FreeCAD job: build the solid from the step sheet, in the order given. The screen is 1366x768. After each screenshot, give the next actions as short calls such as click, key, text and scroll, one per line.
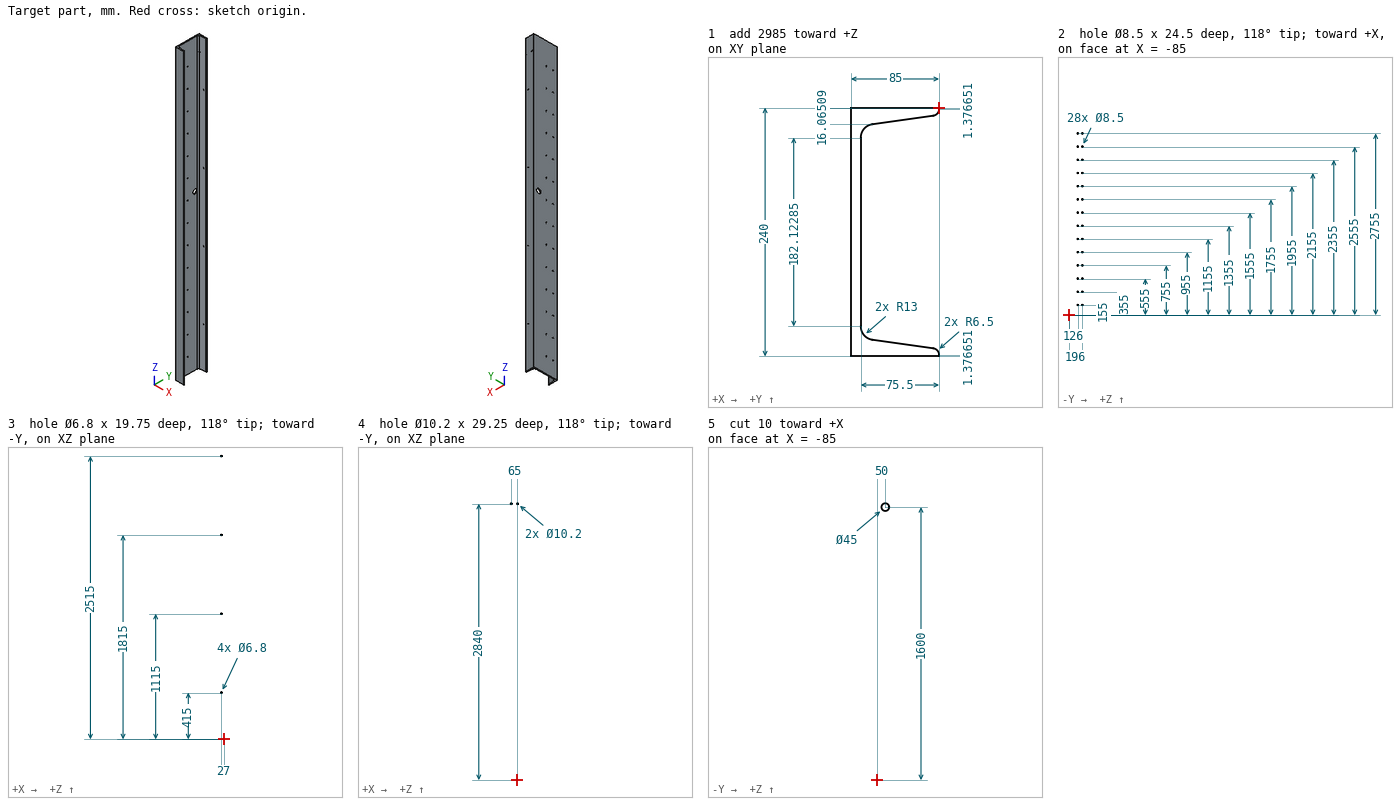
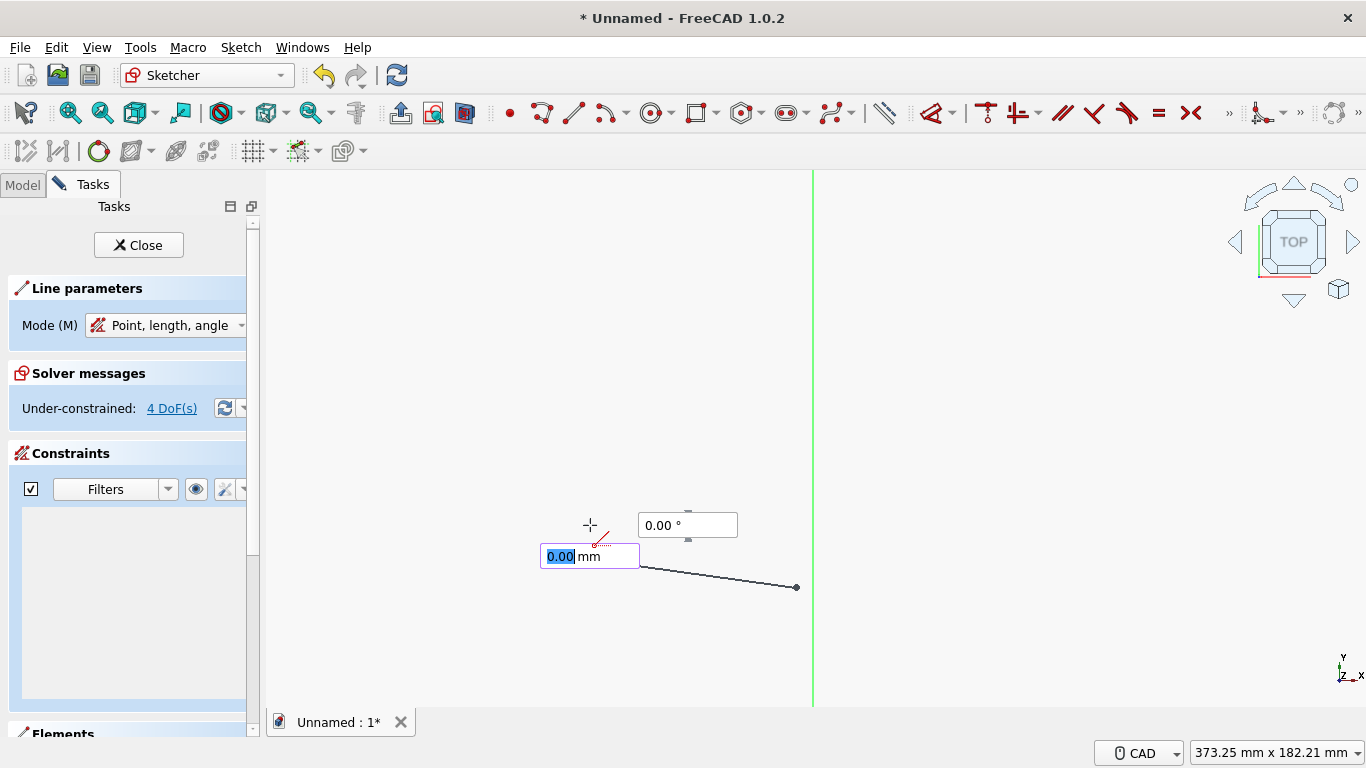
scroll(797, 587, down, 4)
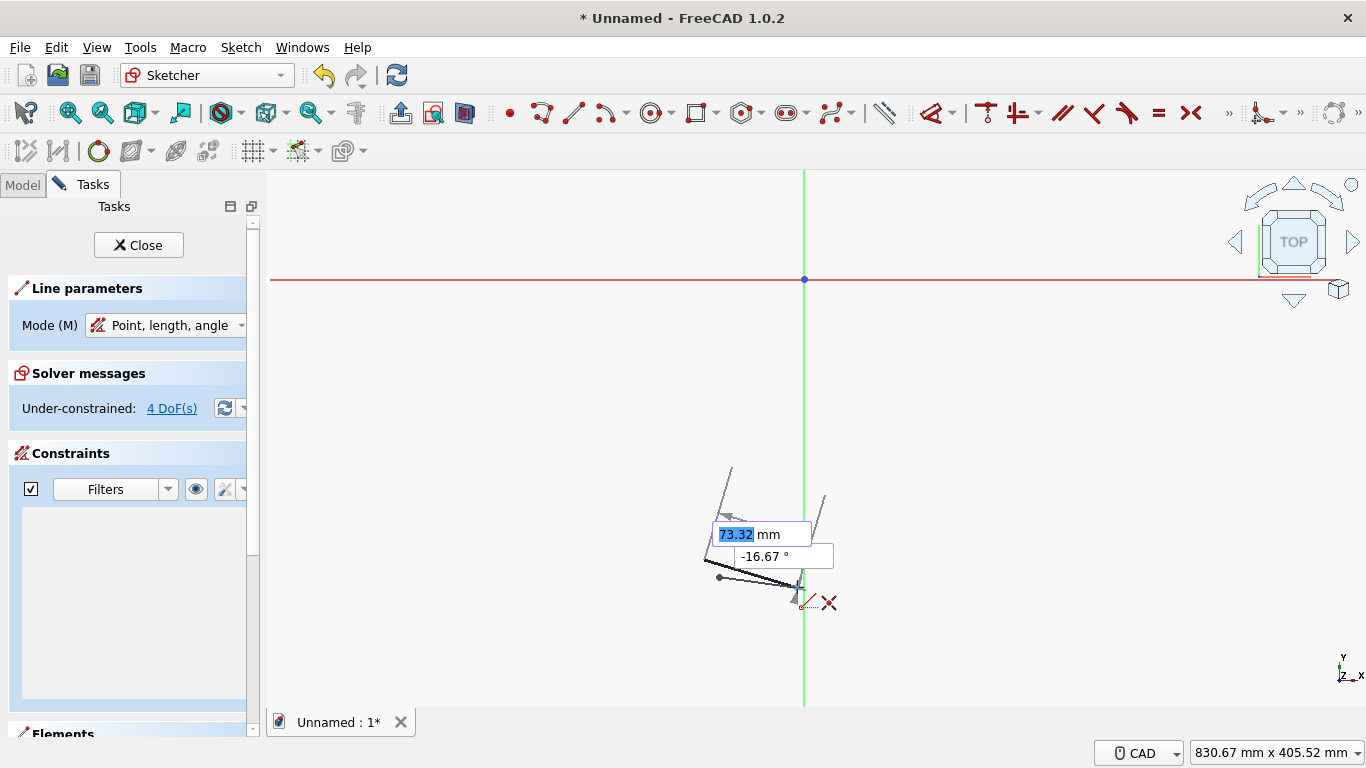
click(704, 318)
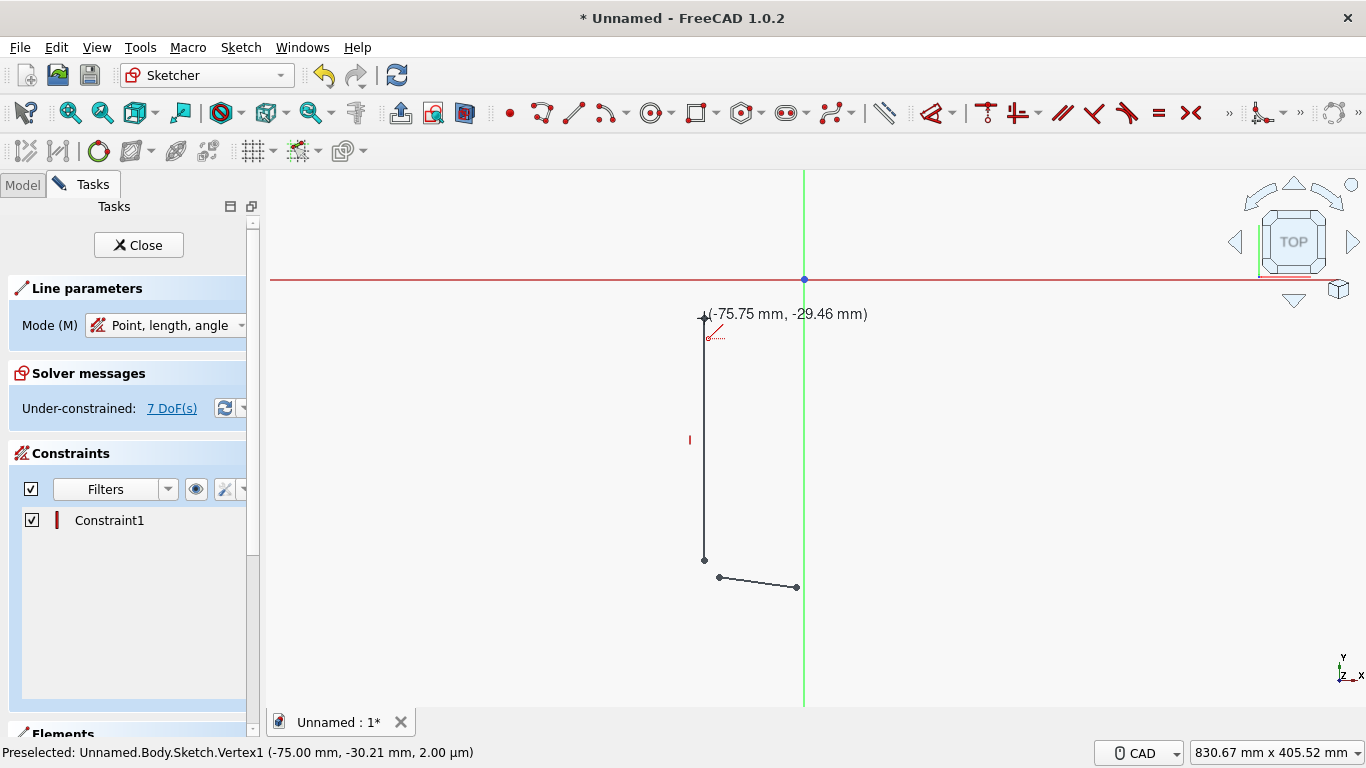
click(719, 301)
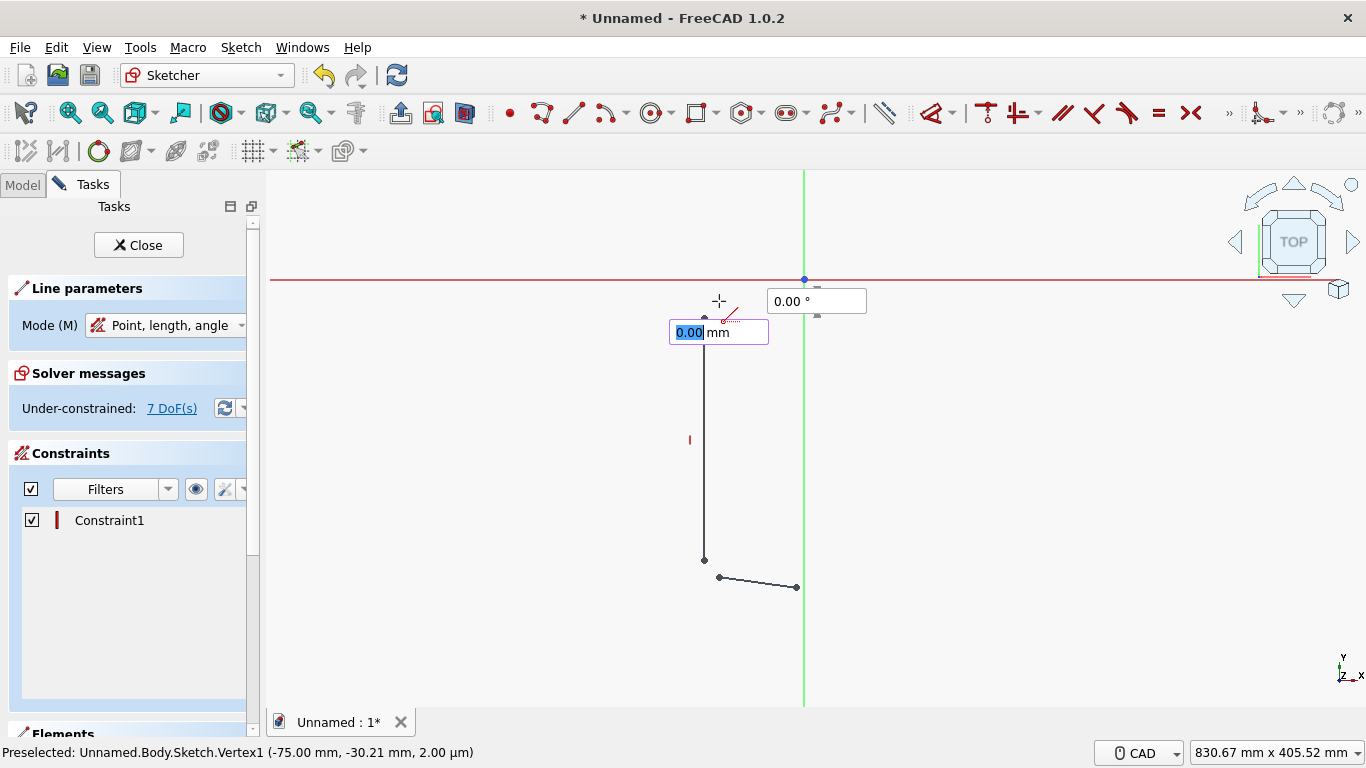
scroll(797, 290, up, 4)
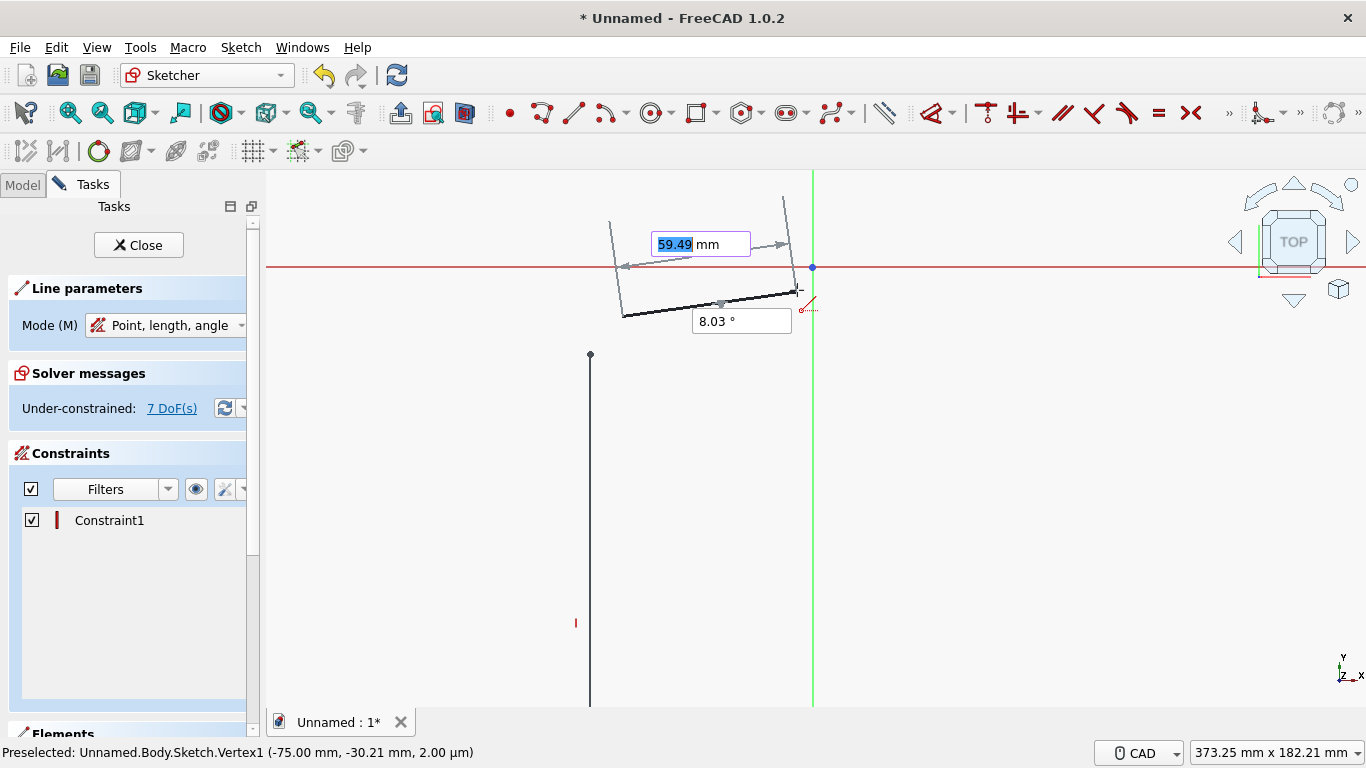
click(796, 290)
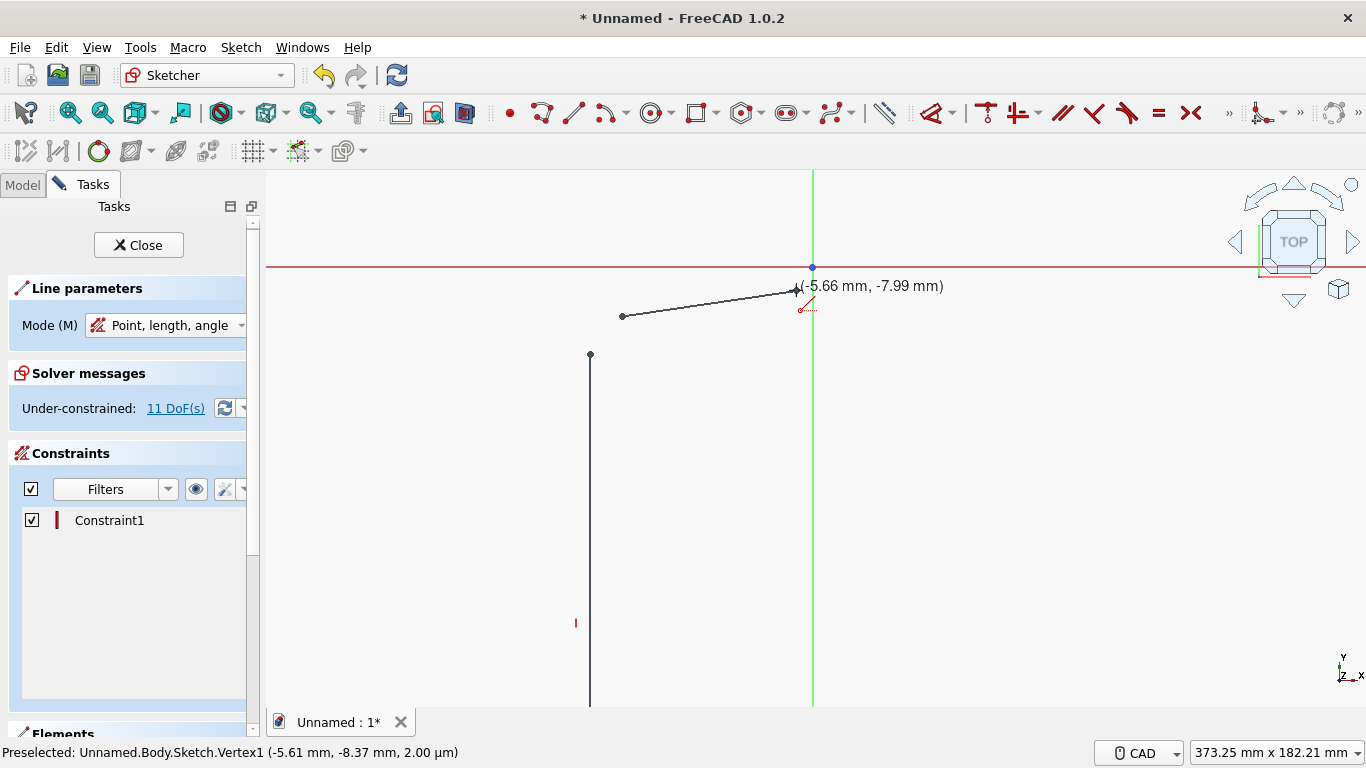
click(542, 114)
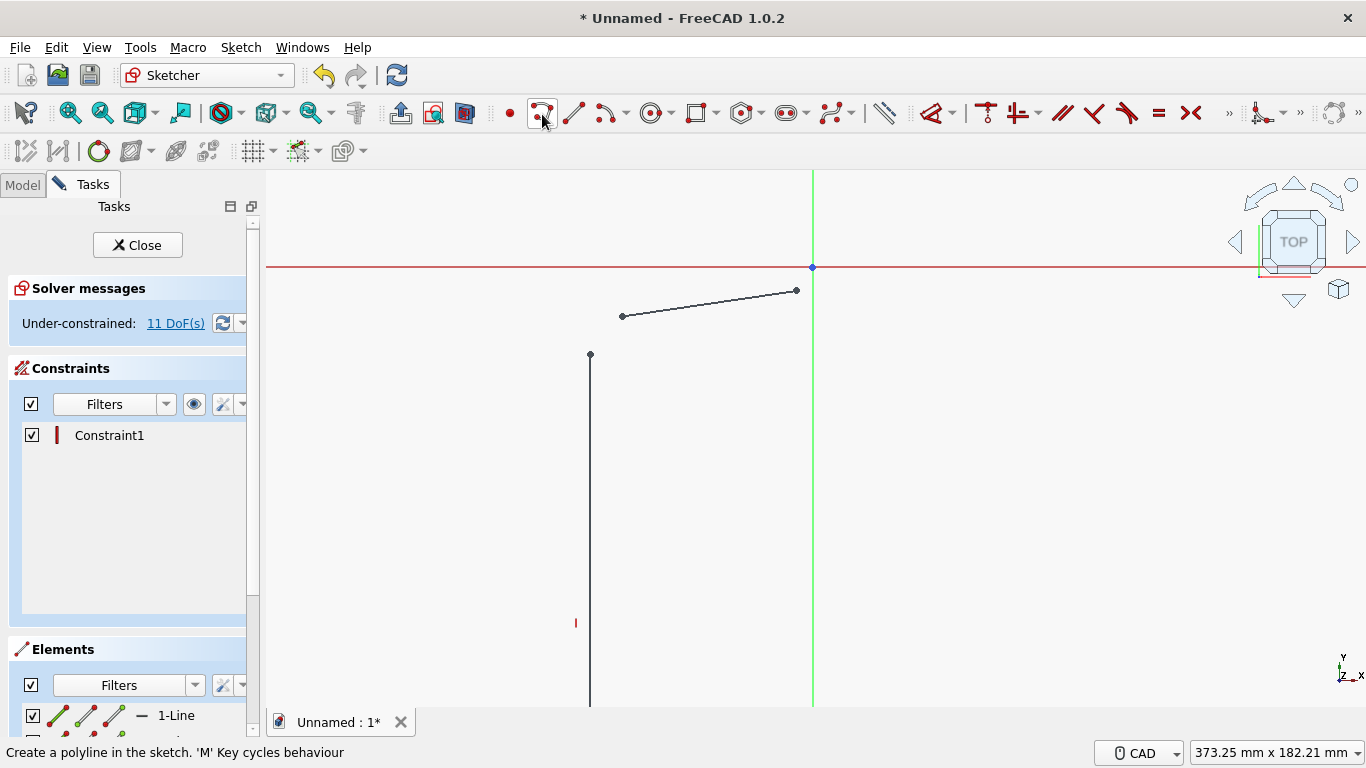
scroll(813, 272, up, 7)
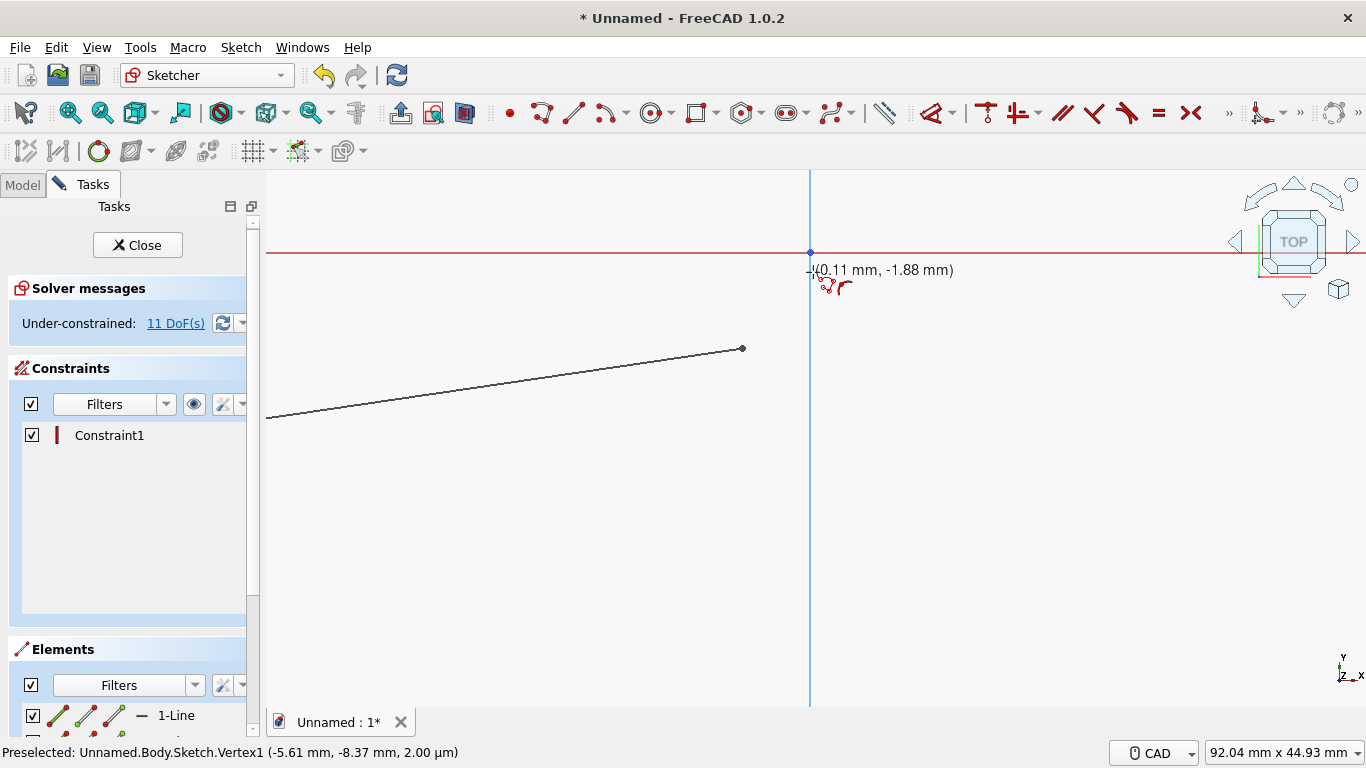
click(810, 269)
click(810, 253)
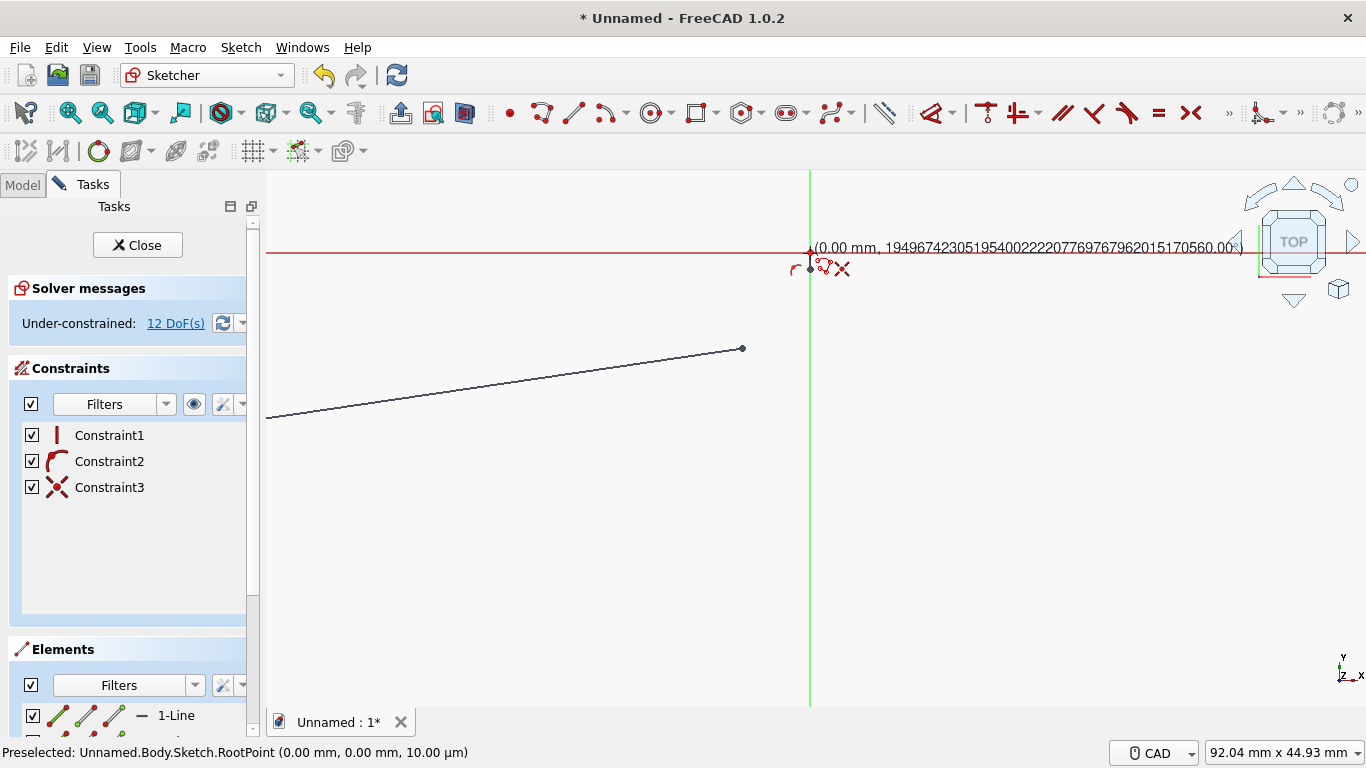
scroll(803, 283, down, 11)